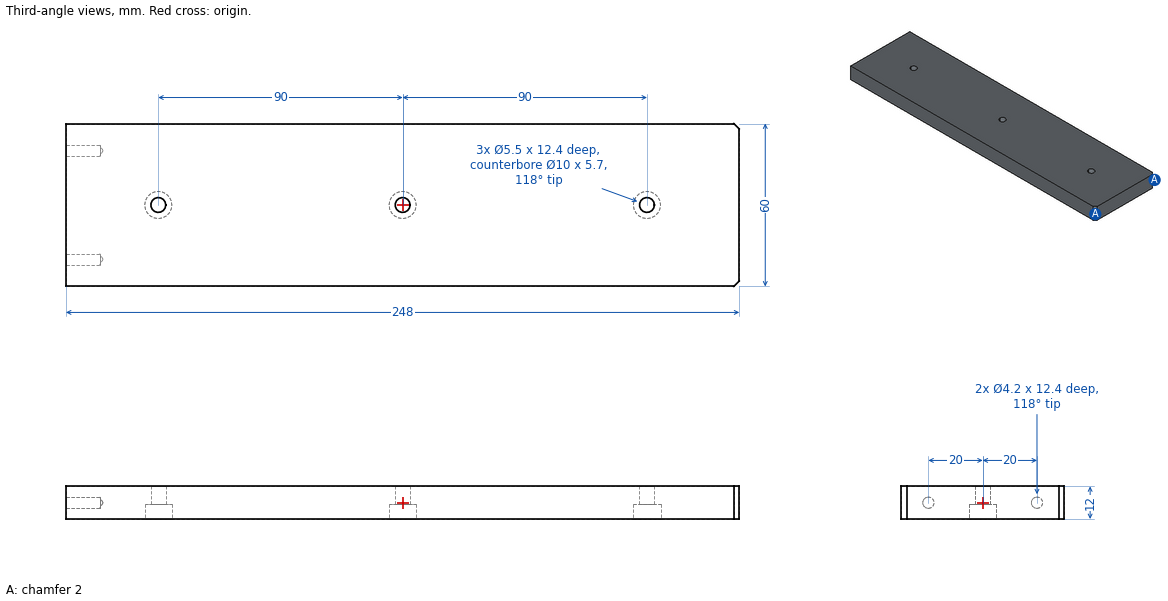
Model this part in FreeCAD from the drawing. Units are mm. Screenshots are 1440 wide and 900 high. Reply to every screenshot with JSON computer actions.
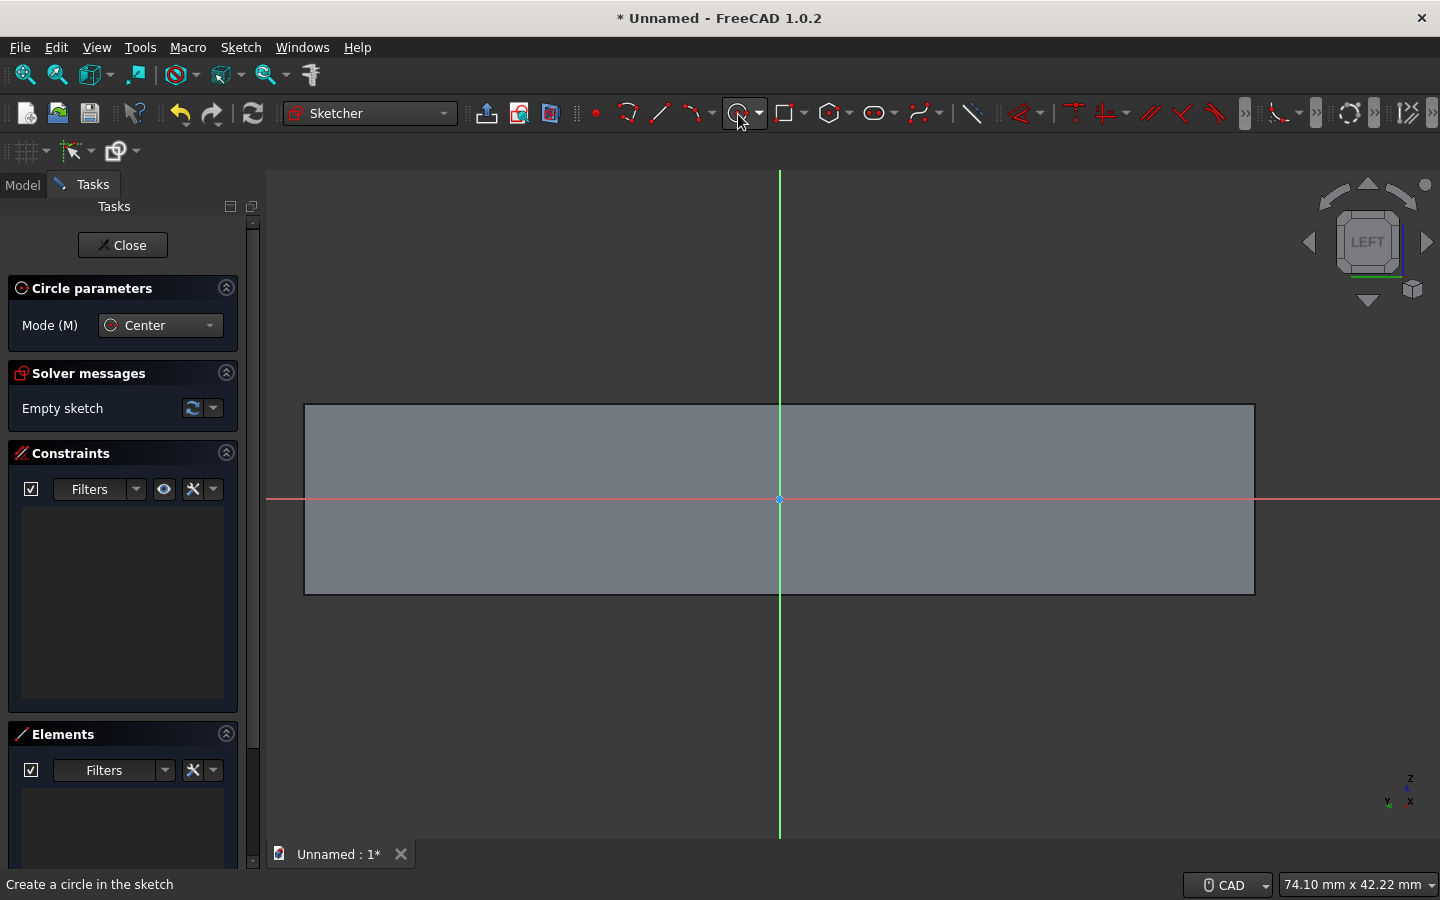
{"action": "left_click", "coordinate": [463, 499]}
{"action": "left_click", "coordinate": [486, 476]}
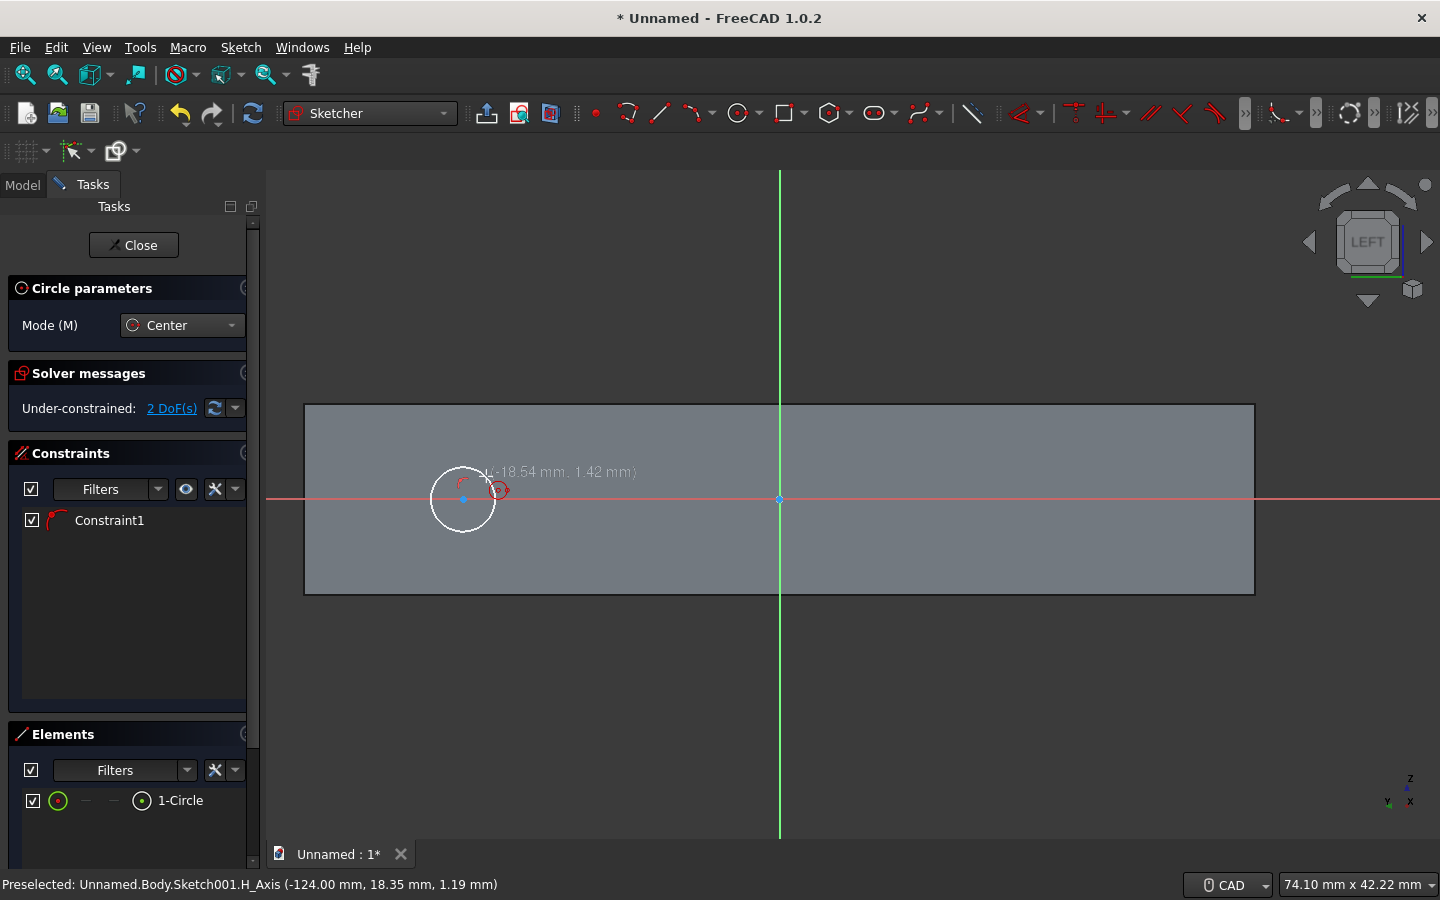
{"action": "left_click", "coordinate": [1097, 499]}
{"action": "left_click", "coordinate": [1120, 476]}
{"action": "key", "text": "Escape"}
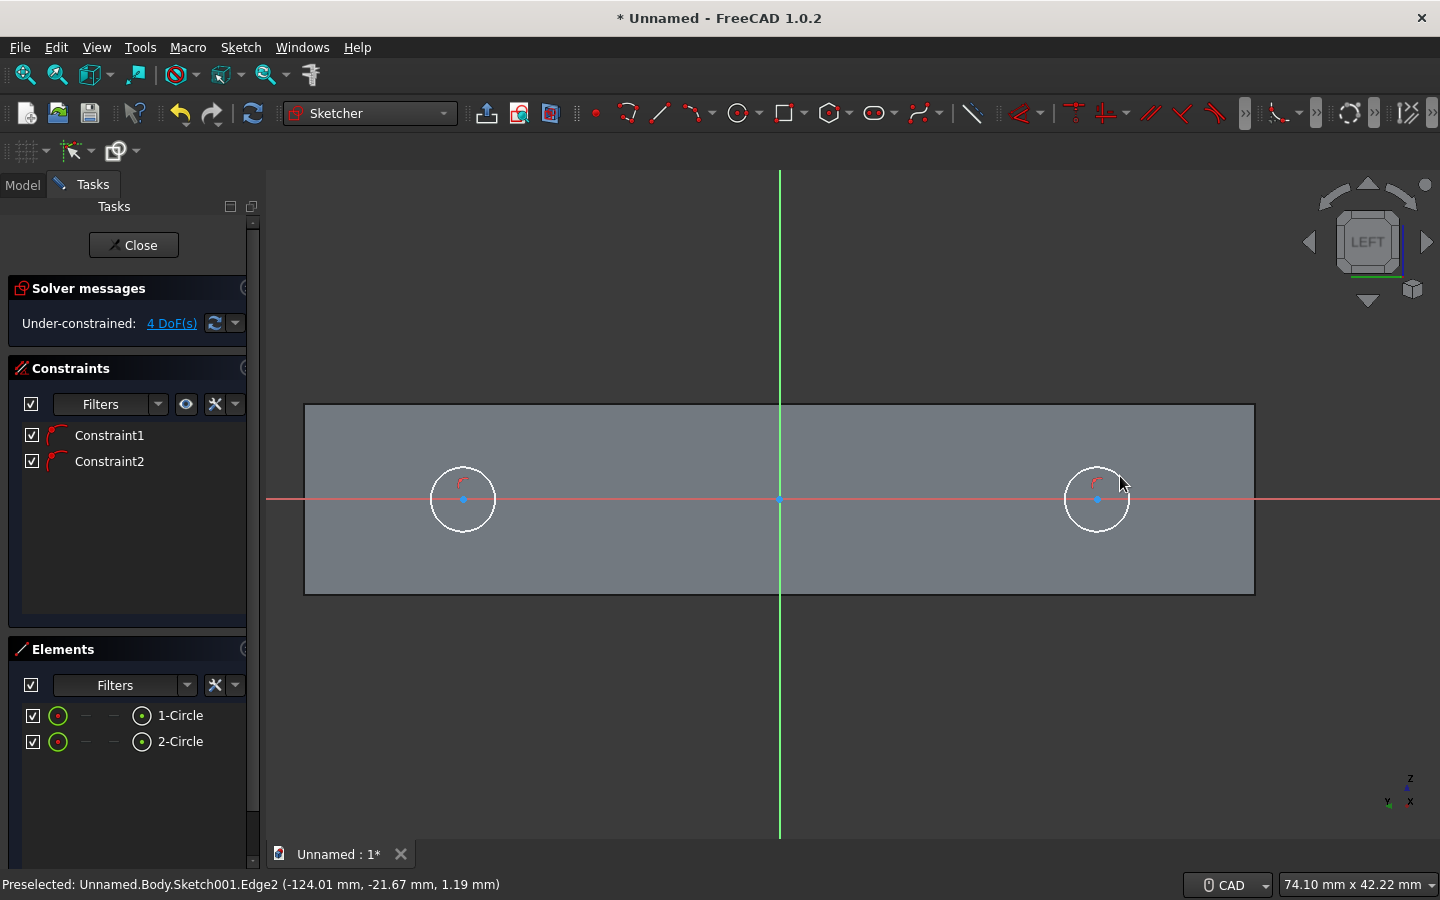
{"action": "left_click", "coordinate": [486, 477]}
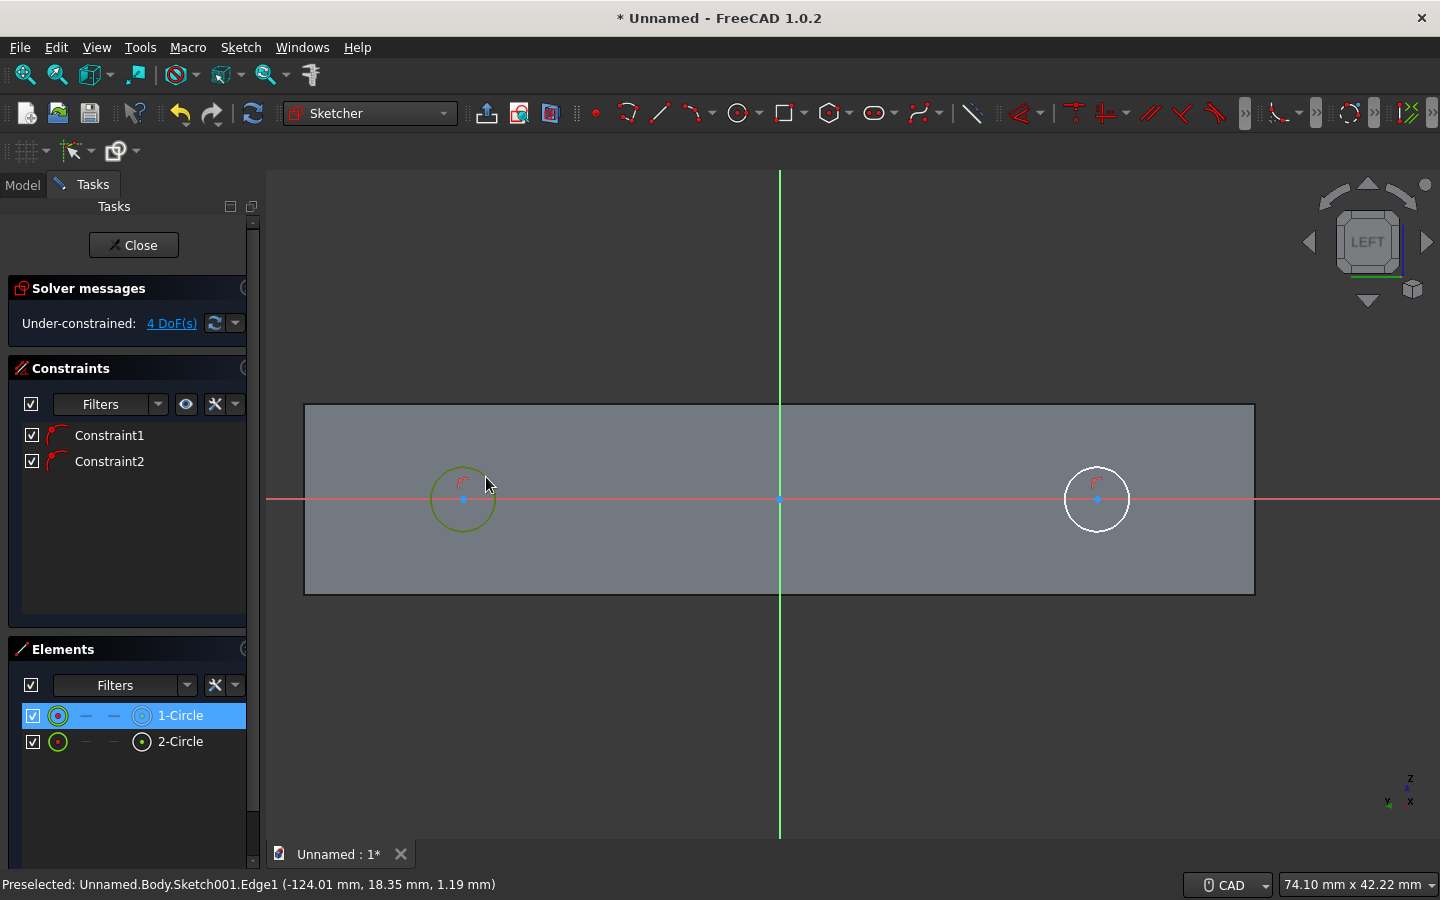
{"action": "left_click", "coordinate": [1120, 477]}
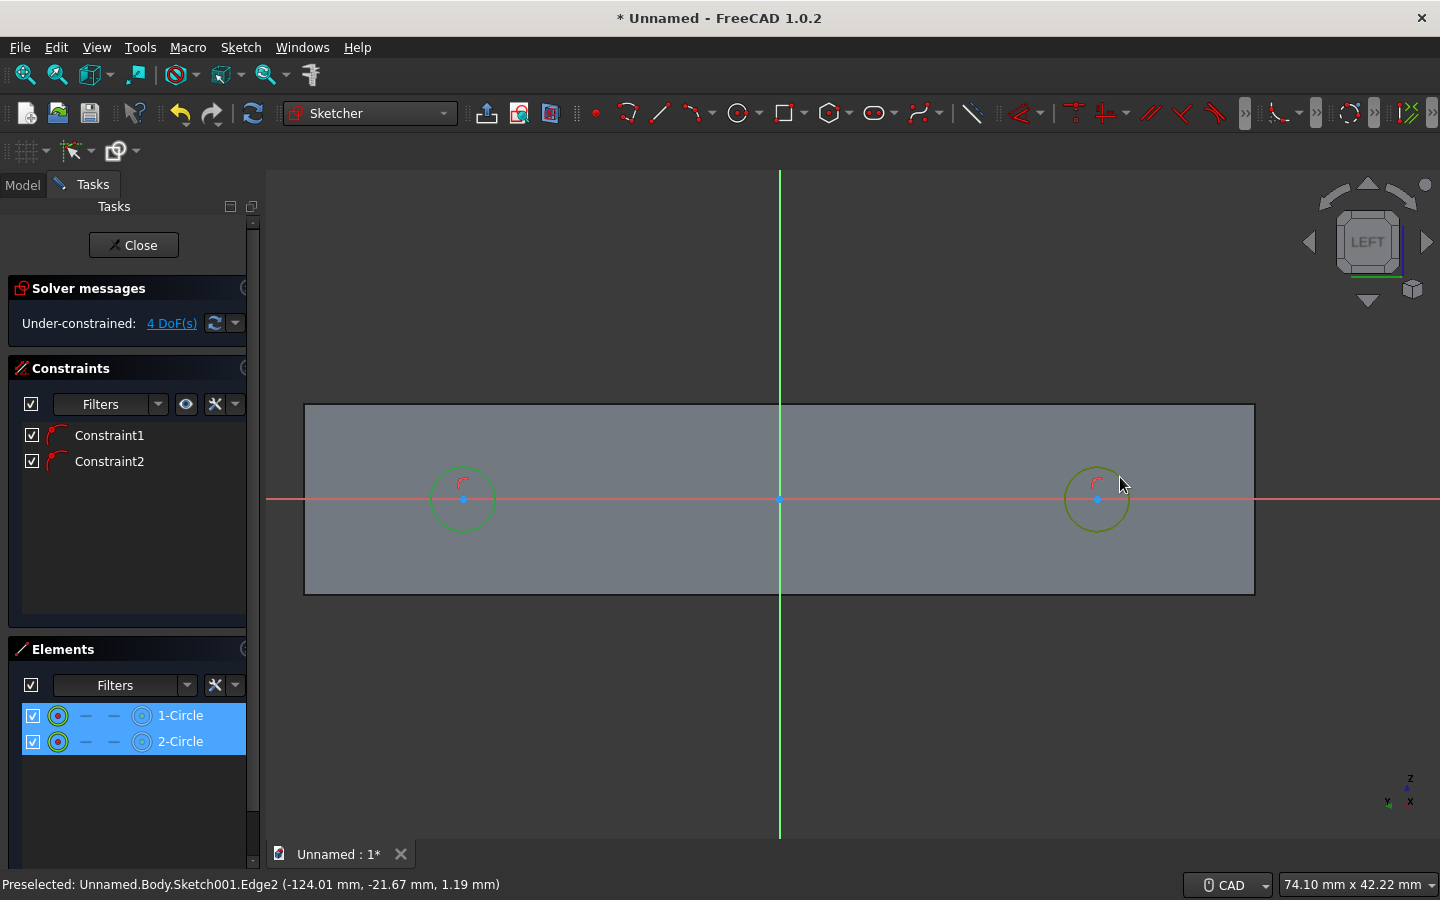
{"action": "key", "text": "e"}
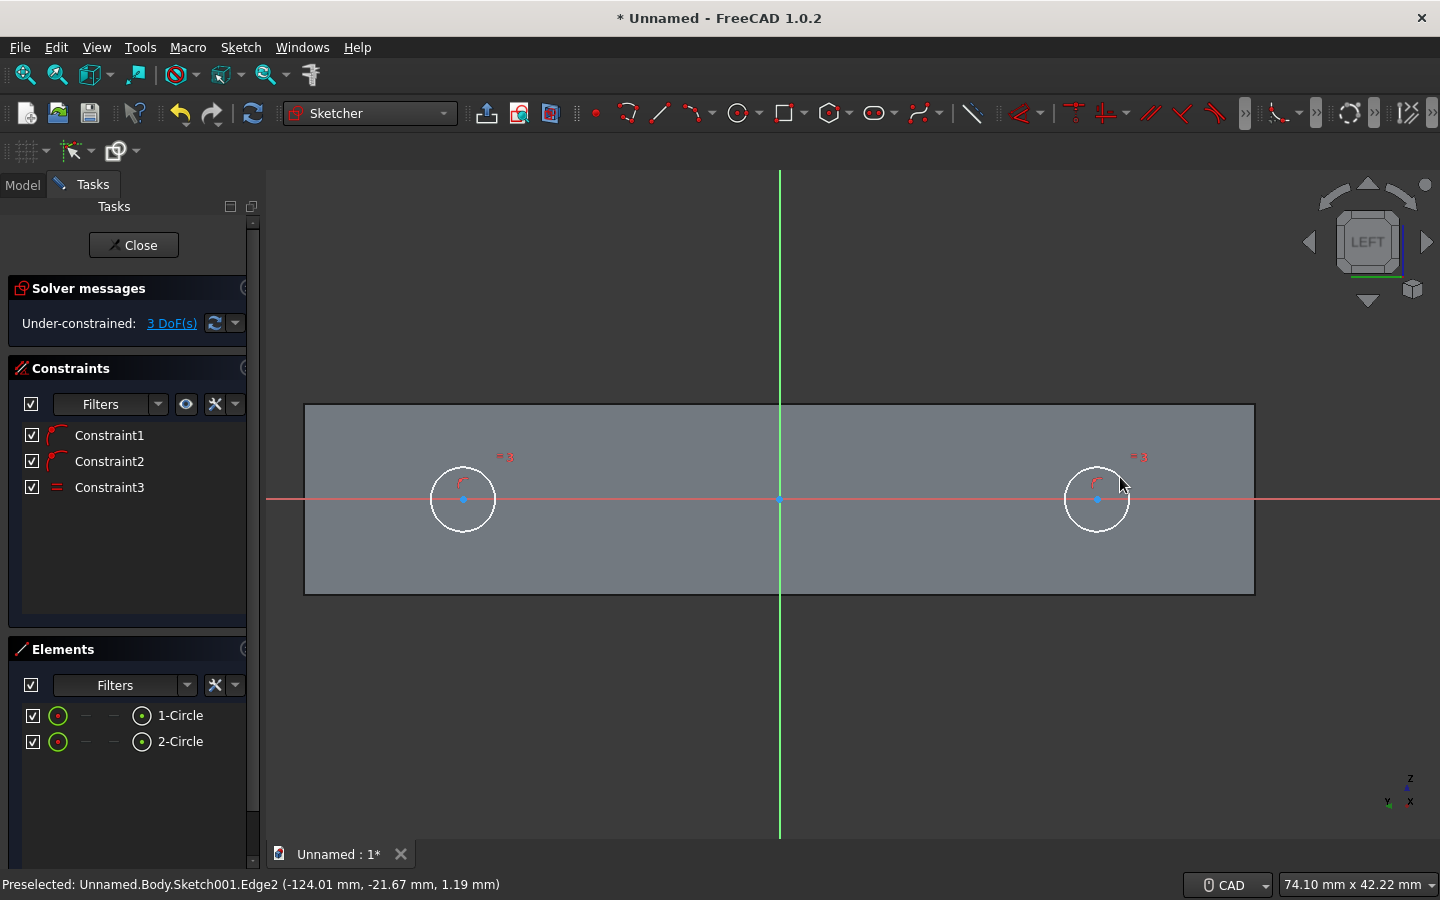
{"action": "left_click", "coordinate": [1020, 114]}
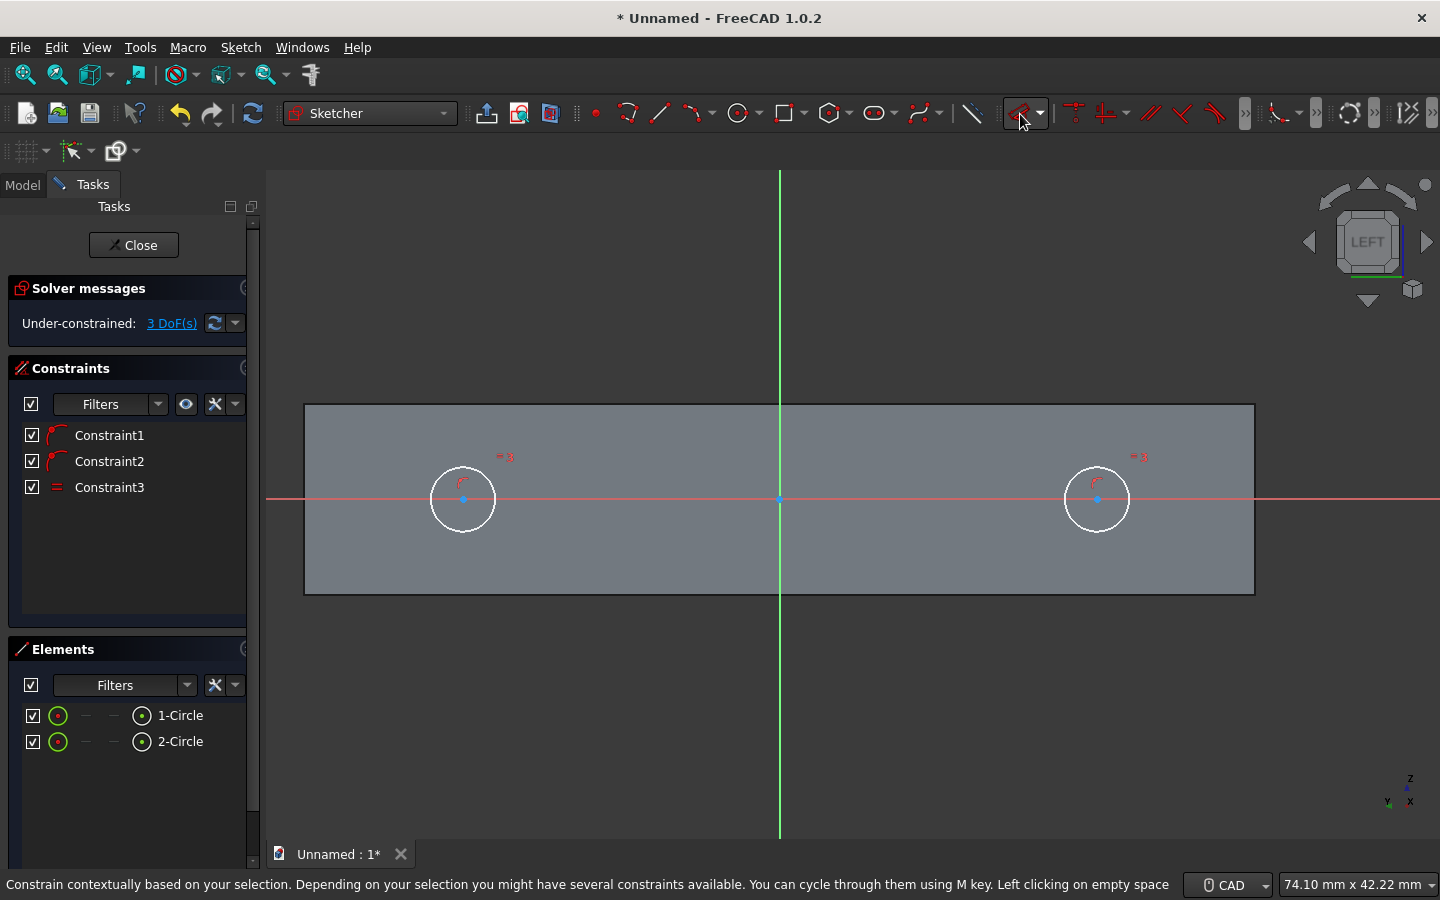
{"action": "left_click", "coordinate": [486, 477]}
{"action": "left_click", "coordinate": [509, 455]}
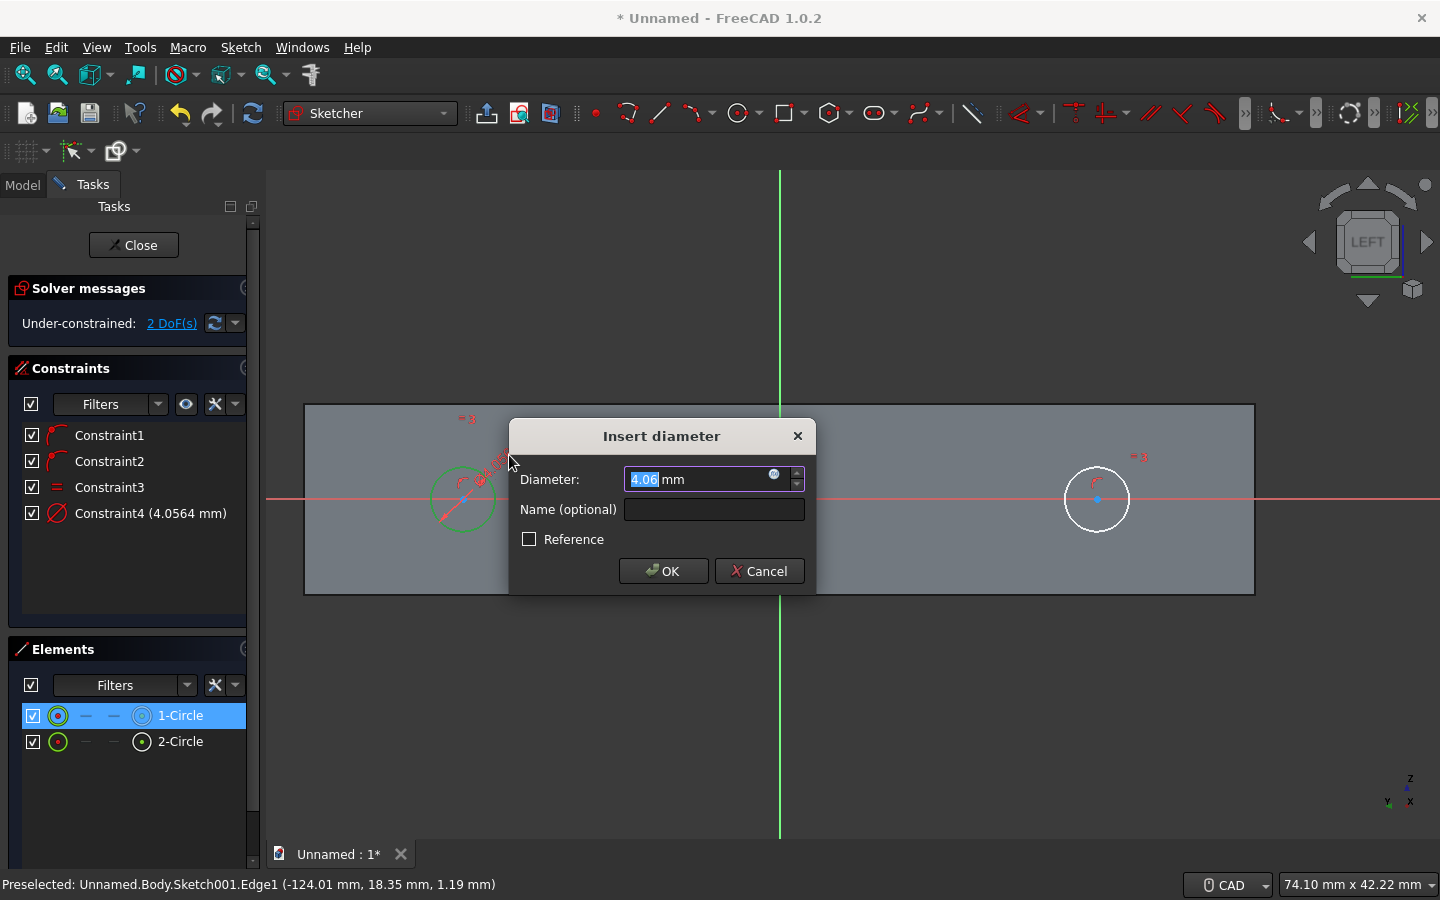
{"action": "type", "text": "4.2"}
{"action": "key", "text": "Return"}